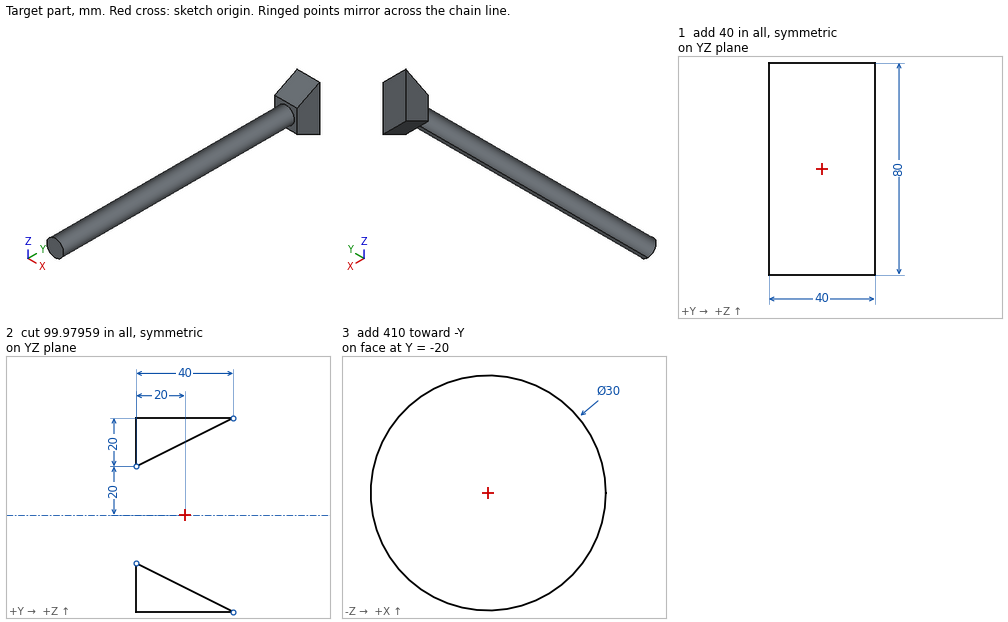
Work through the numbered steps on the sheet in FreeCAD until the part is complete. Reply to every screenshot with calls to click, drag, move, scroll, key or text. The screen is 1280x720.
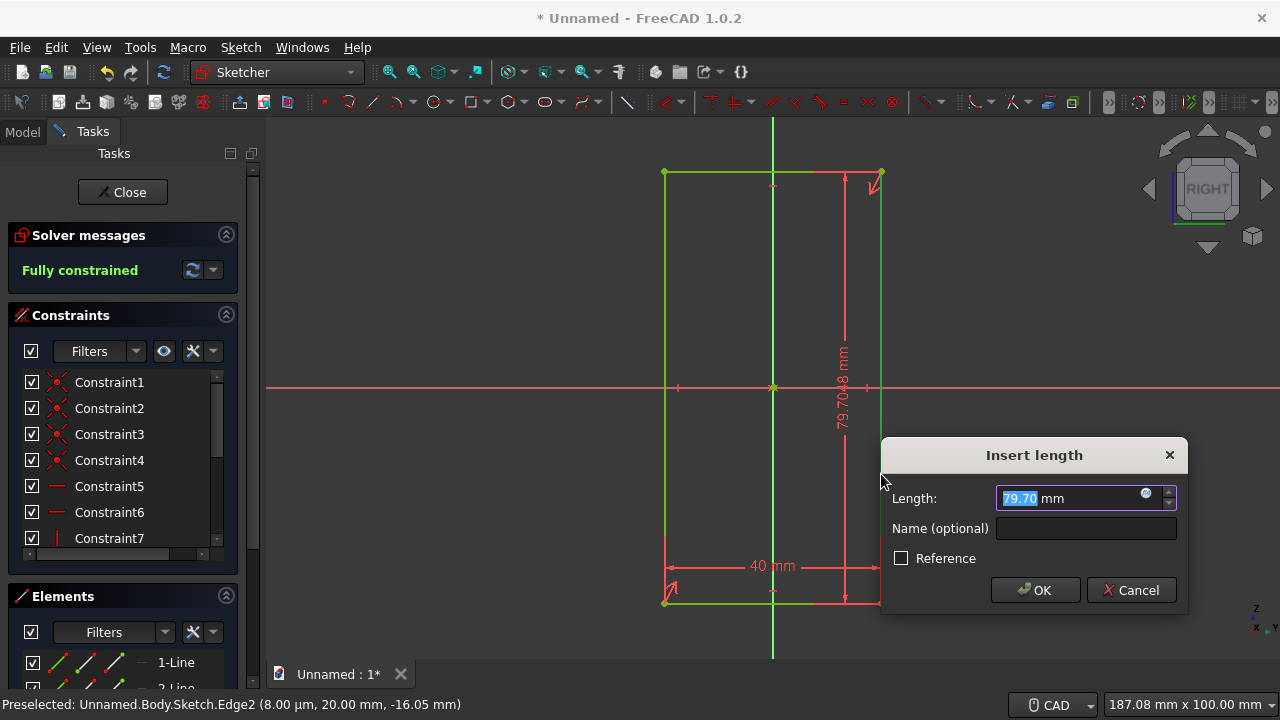
text(80)
key(Return)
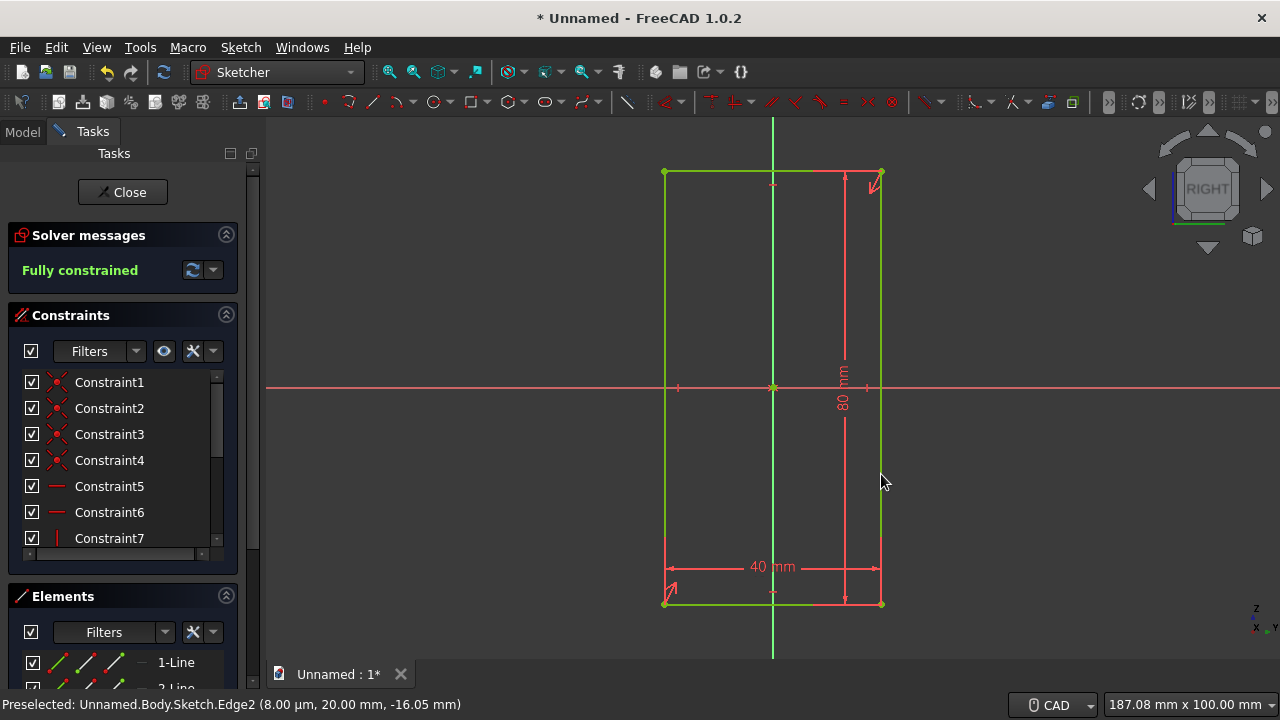
click(123, 192)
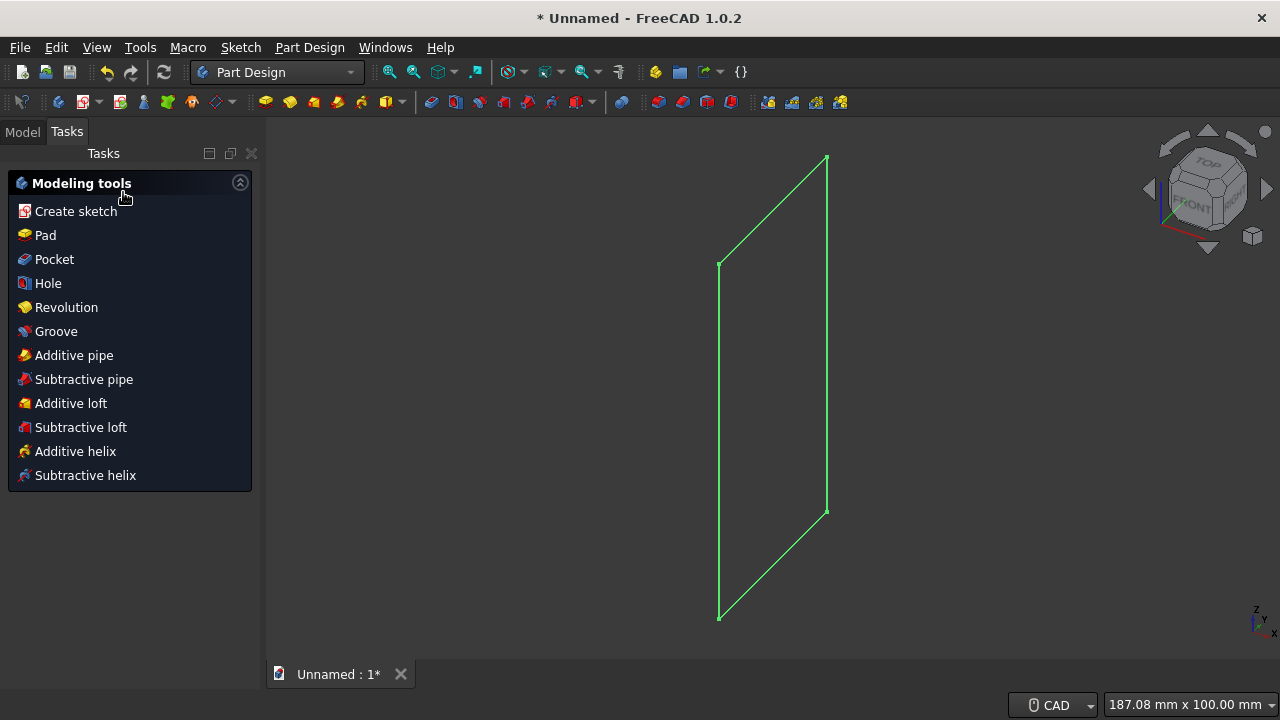
click(266, 102)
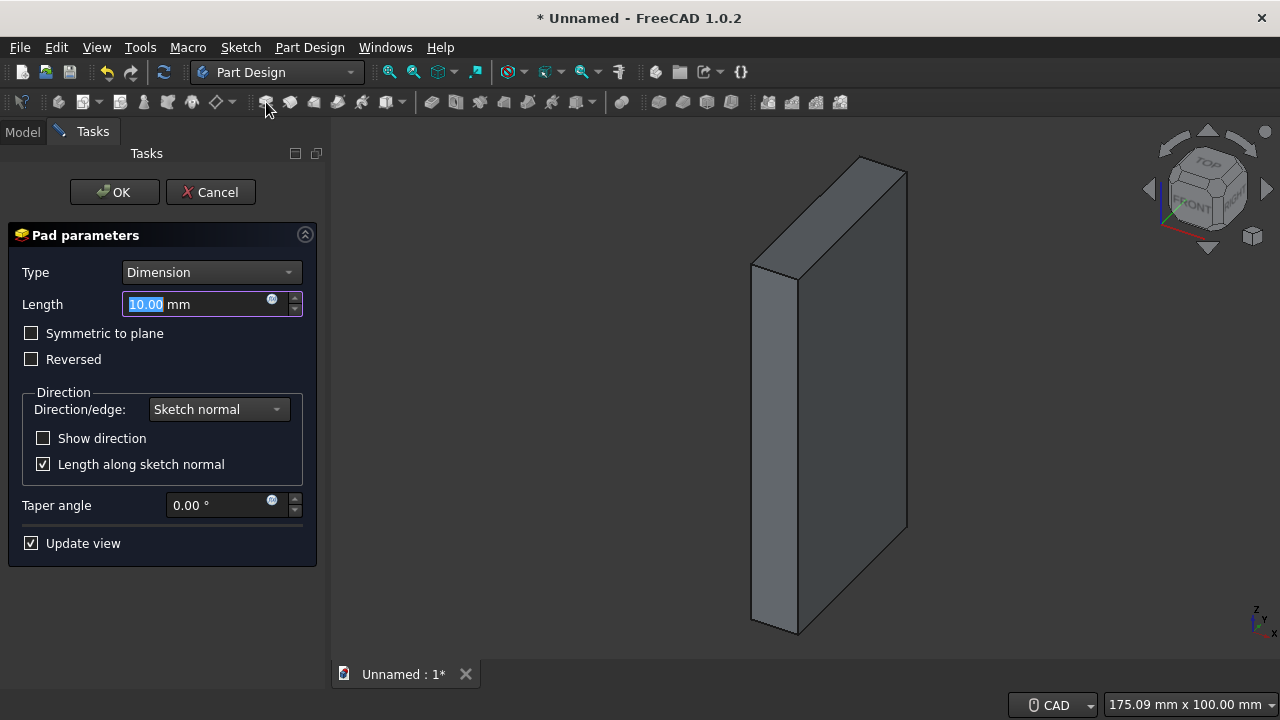
text(40)
key(Tab)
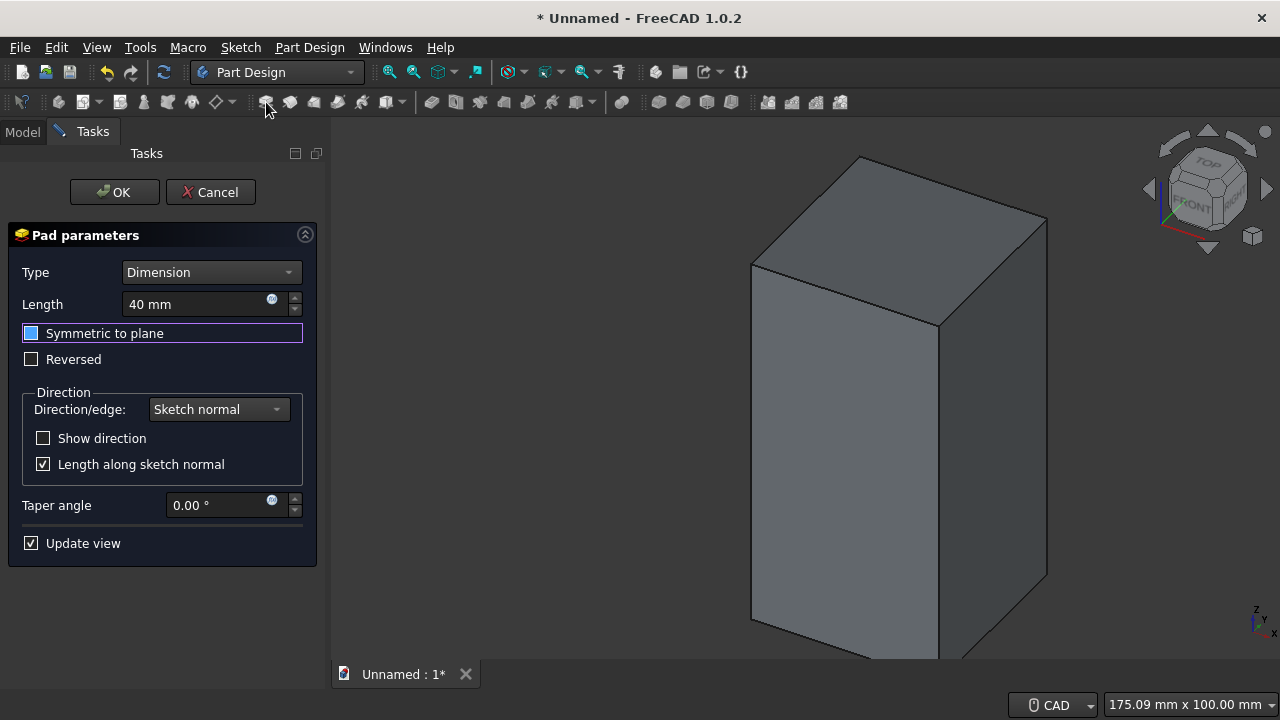
click(30, 333)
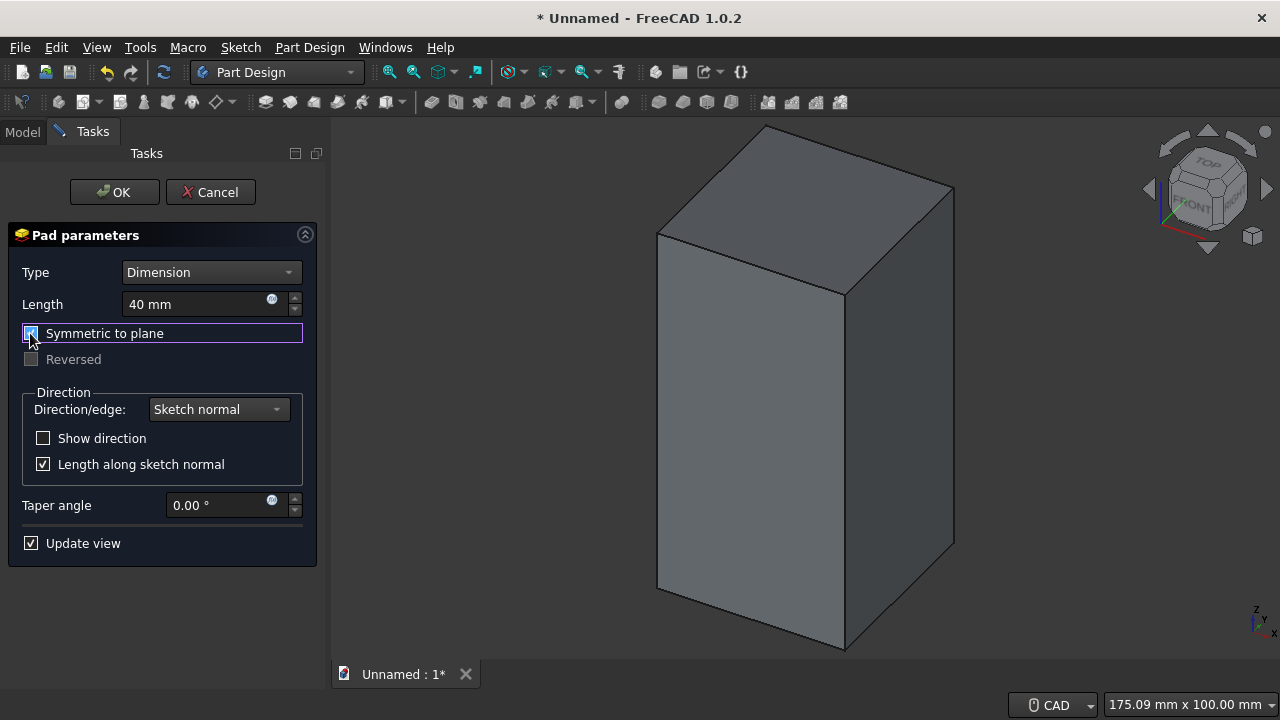
click(115, 192)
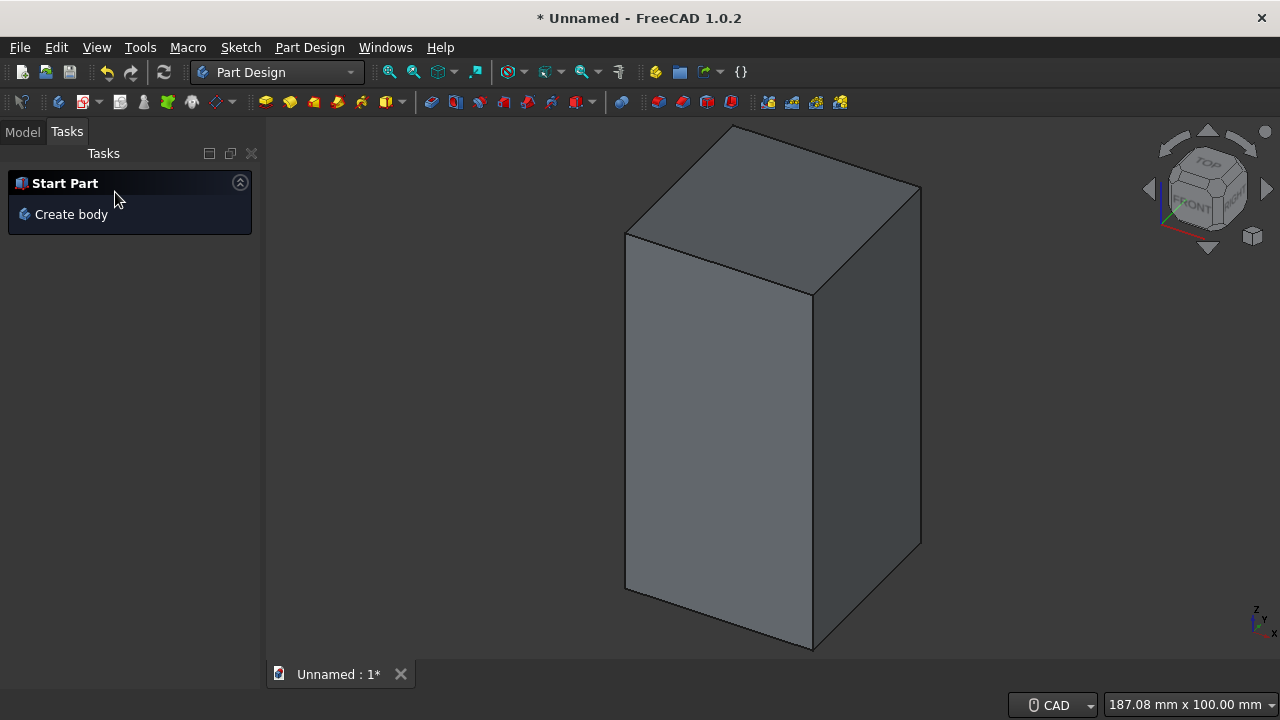
click(84, 102)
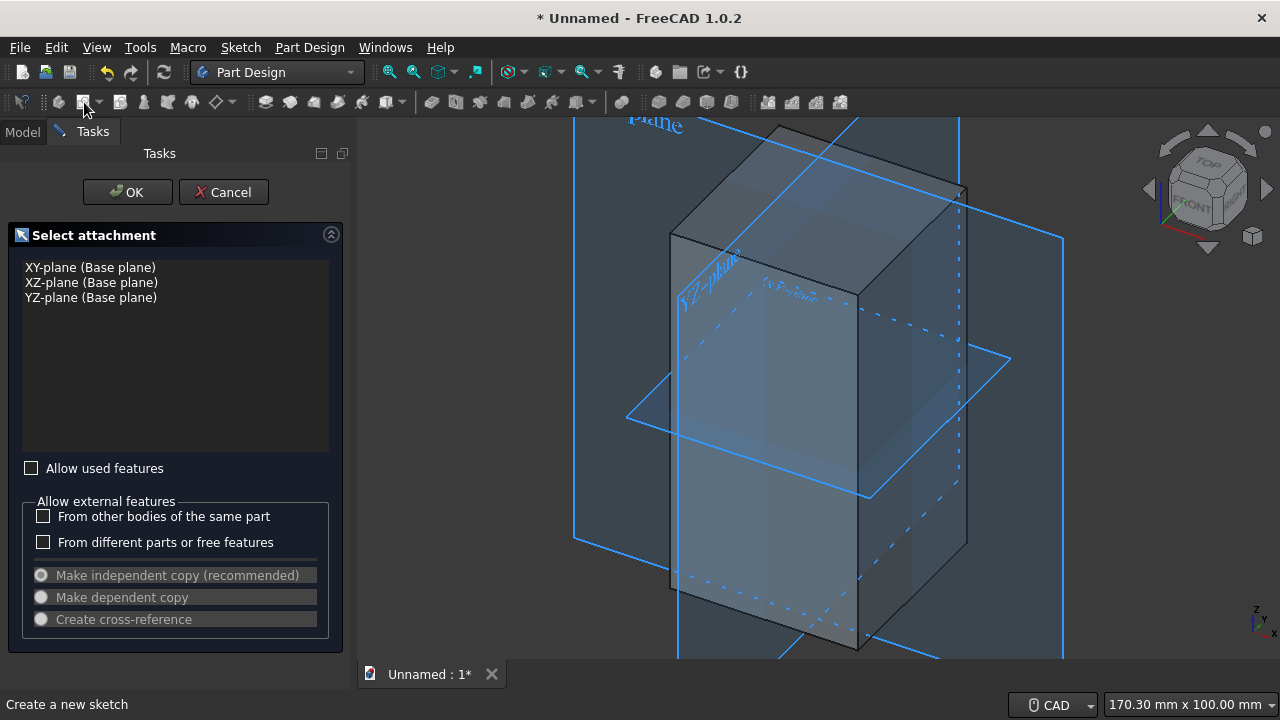
click(82, 298)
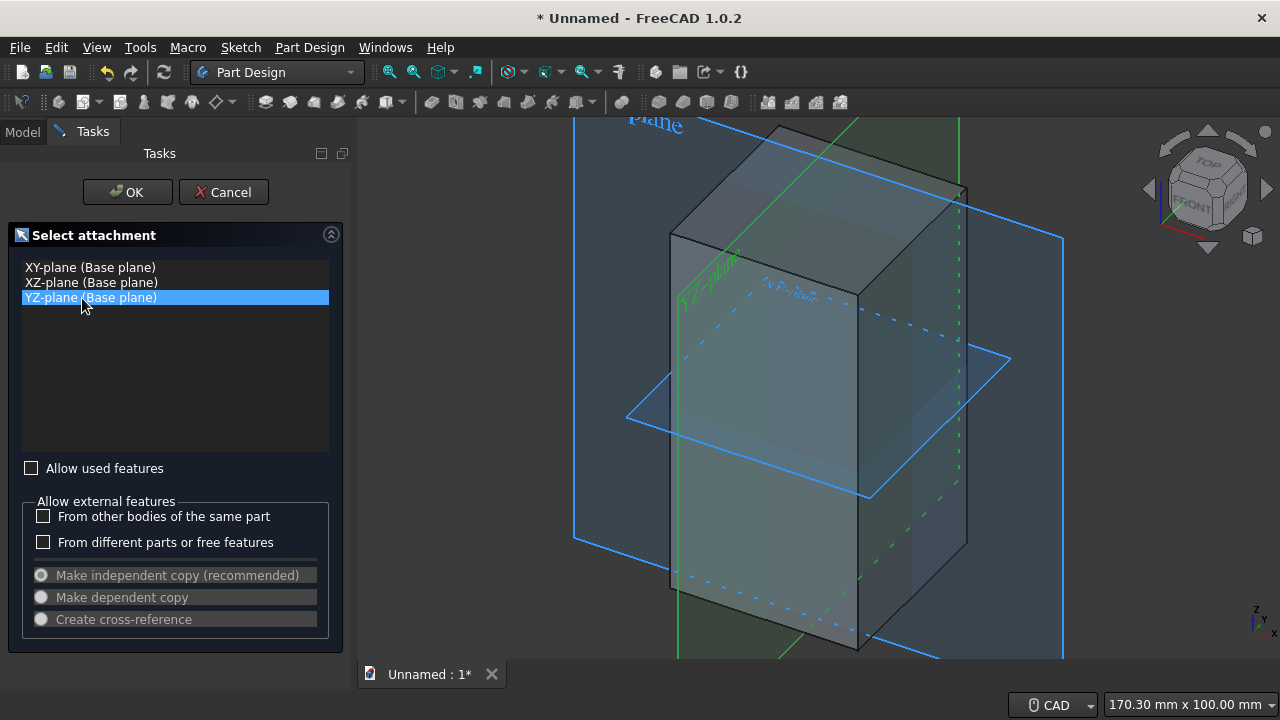
click(128, 192)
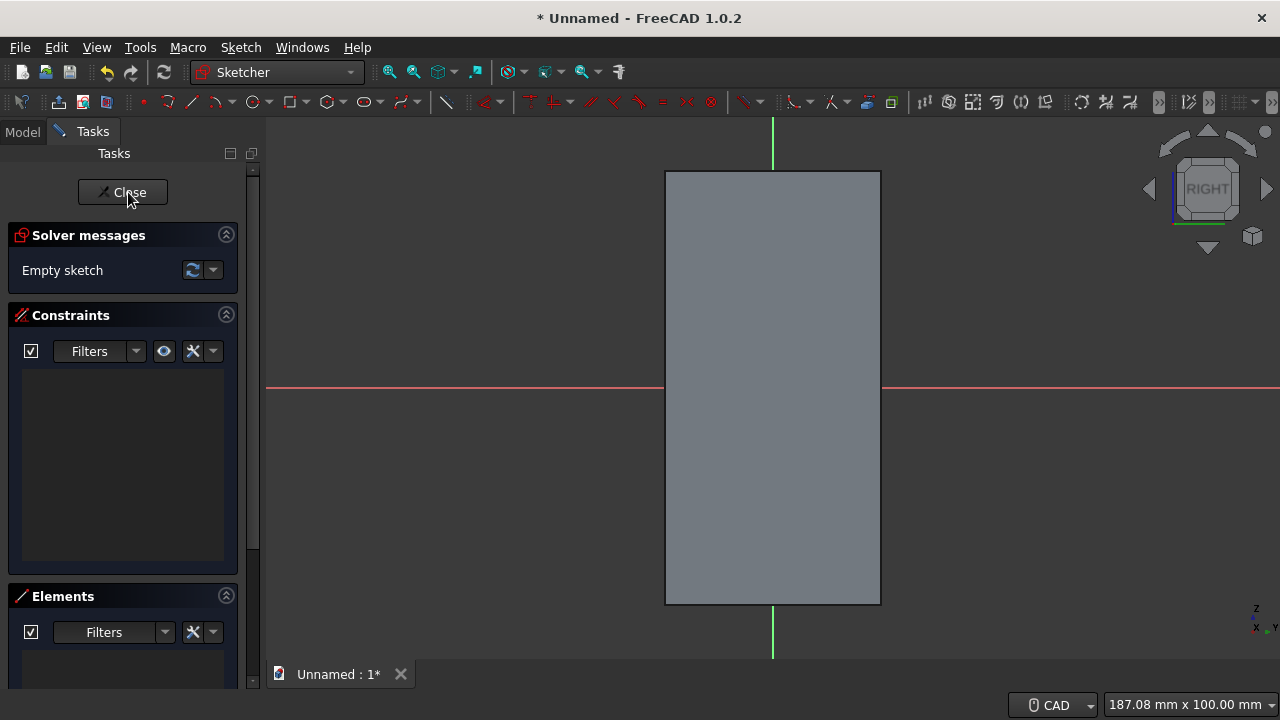
click(108, 102)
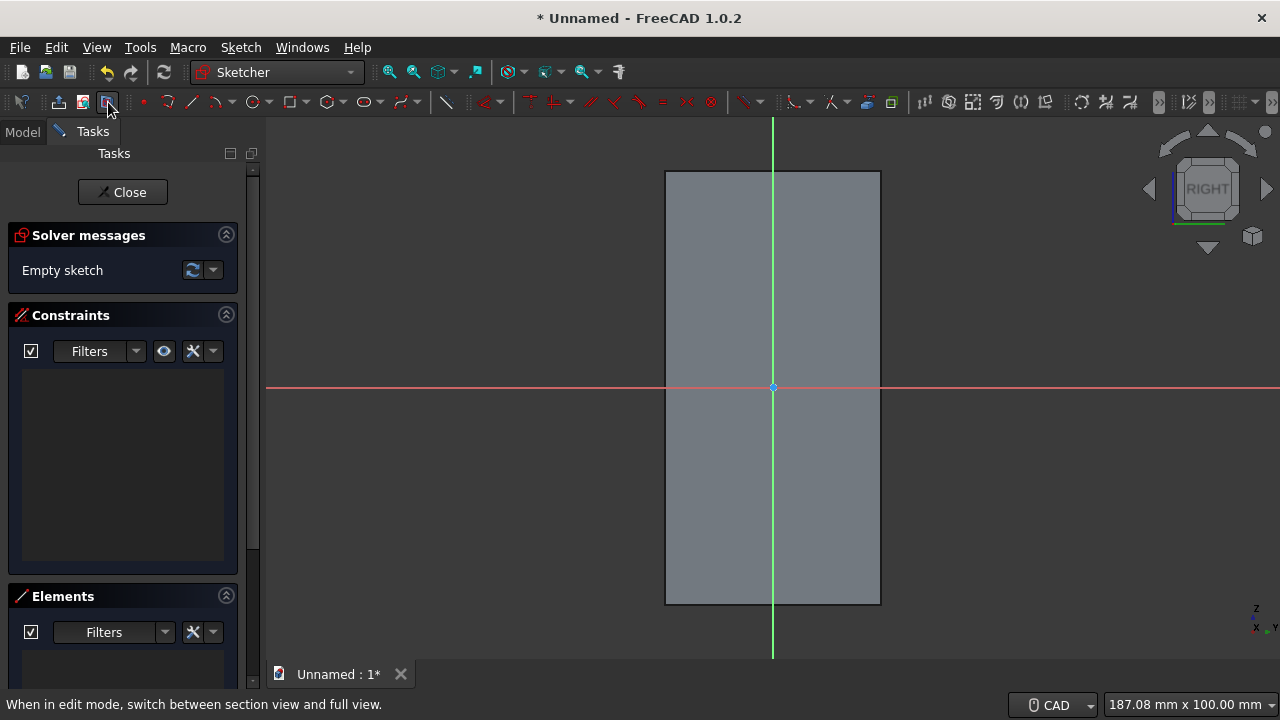
key(g)
key(m)